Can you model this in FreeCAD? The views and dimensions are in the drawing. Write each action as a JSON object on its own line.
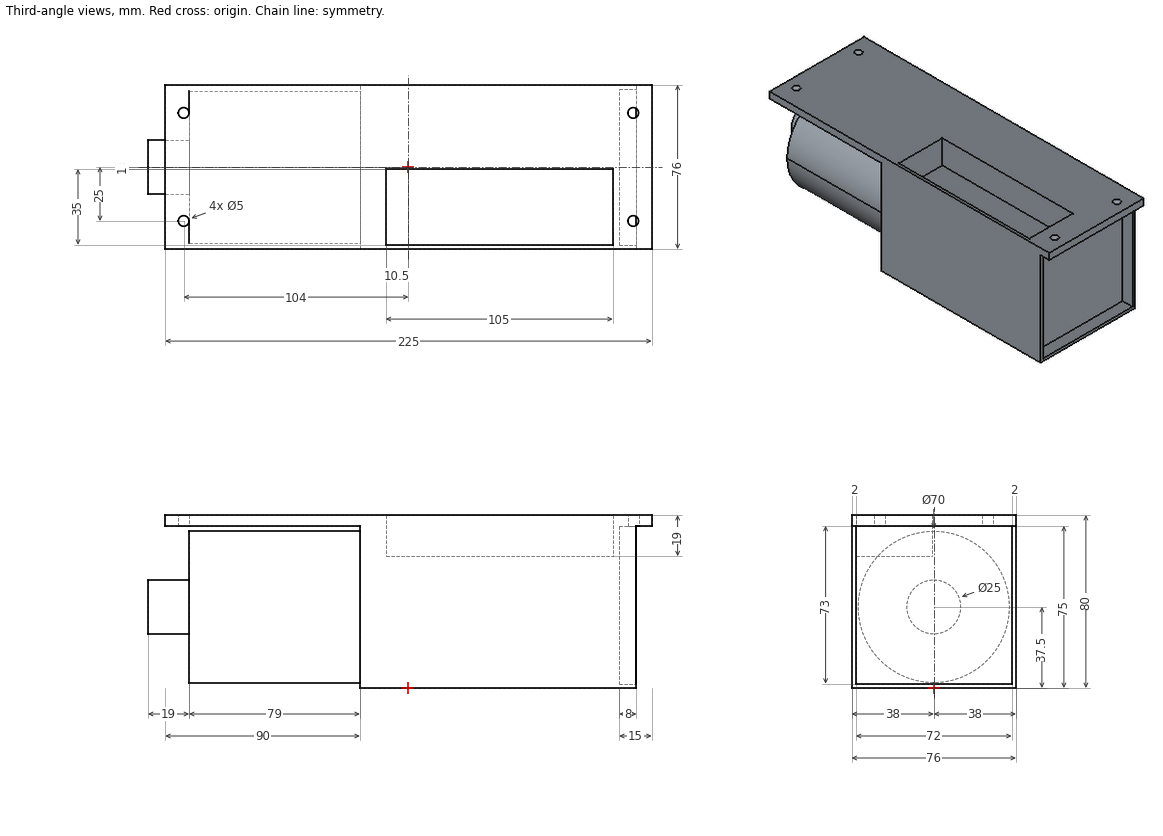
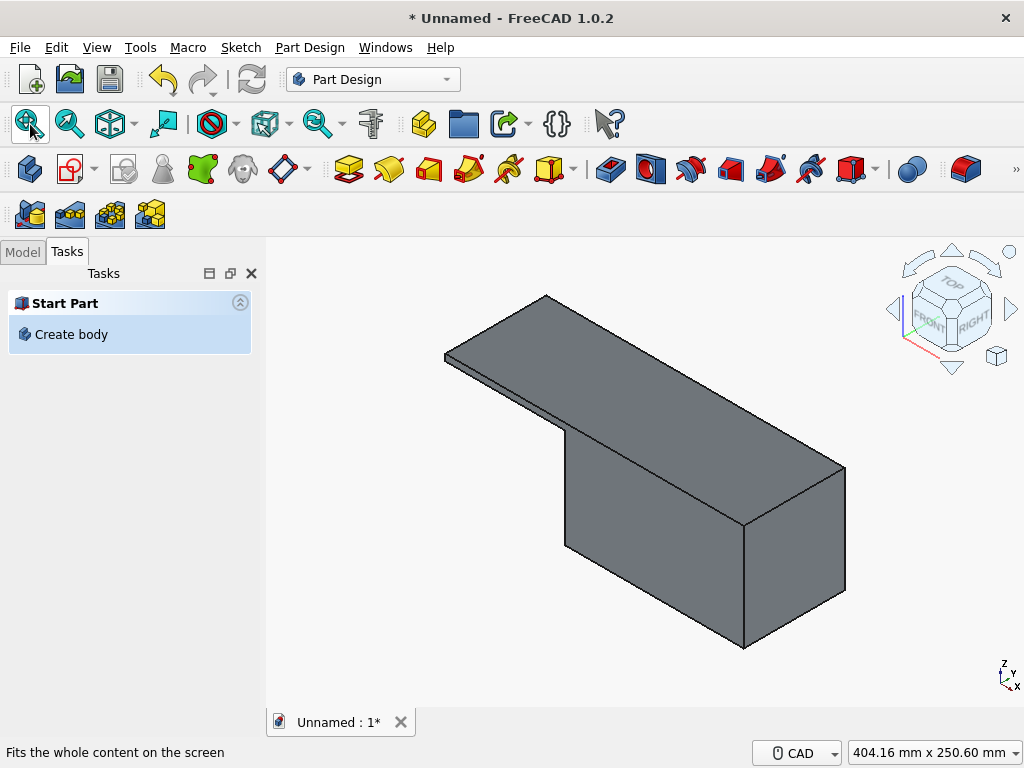
{"action": "left_click", "coordinate": [794, 557]}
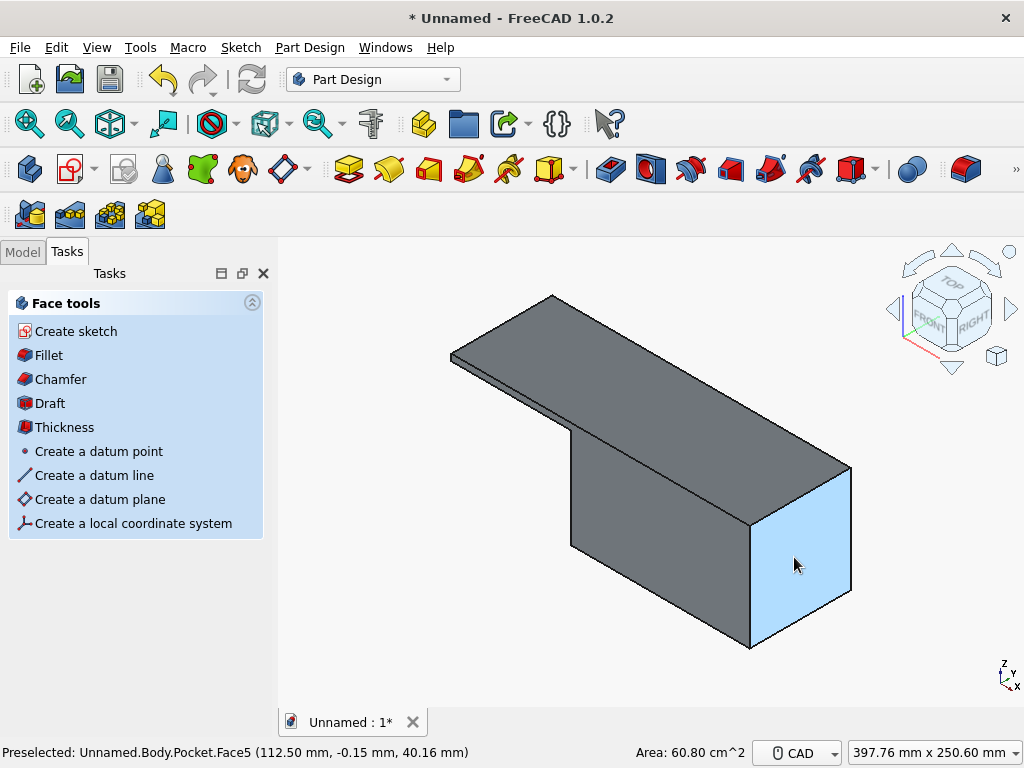
{"action": "left_click", "coordinate": [70, 170]}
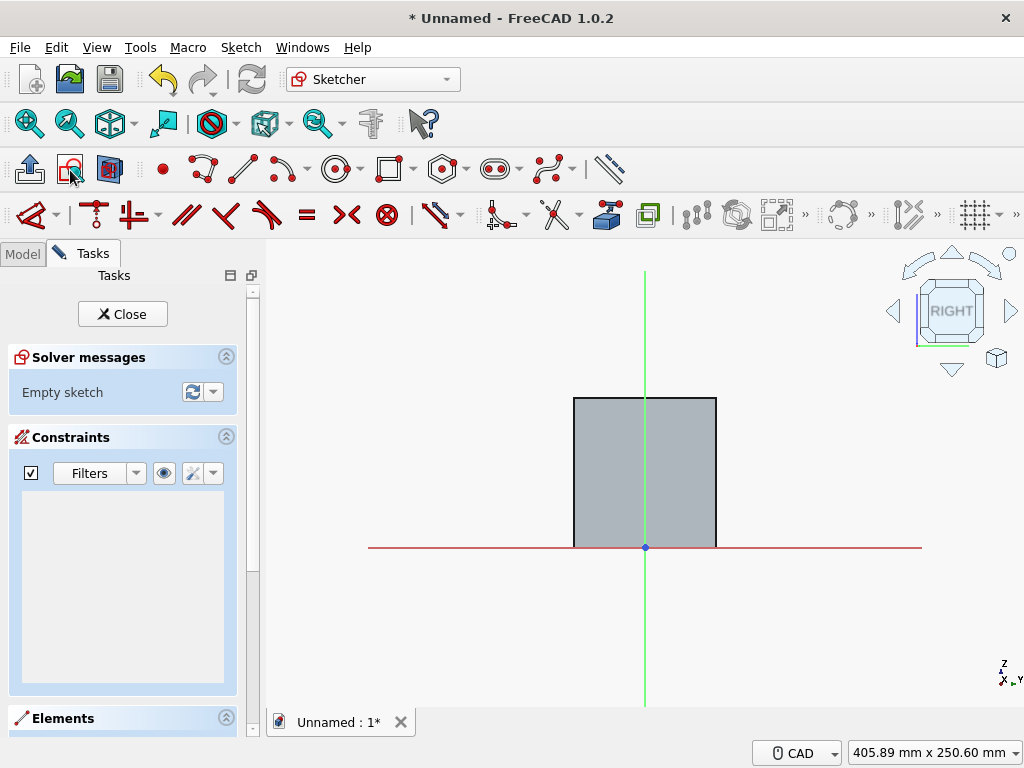
{"action": "scroll", "coordinate": [701, 481], "scroll_direction": "up", "scroll_amount": 4}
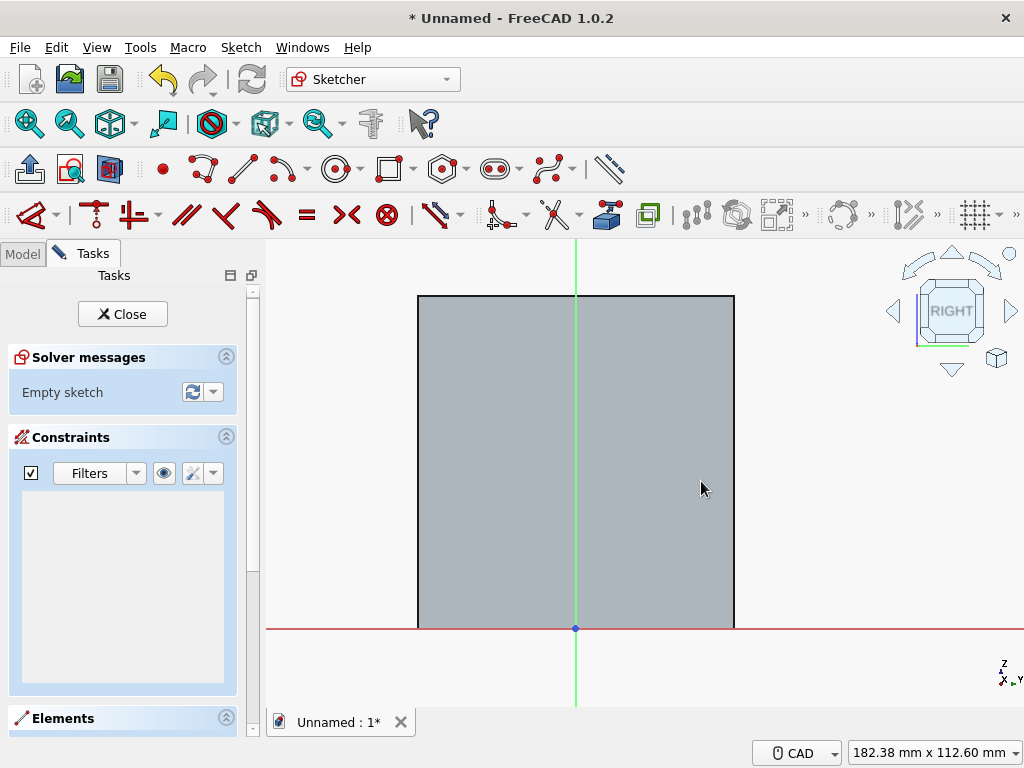
{"action": "key", "text": "g r"}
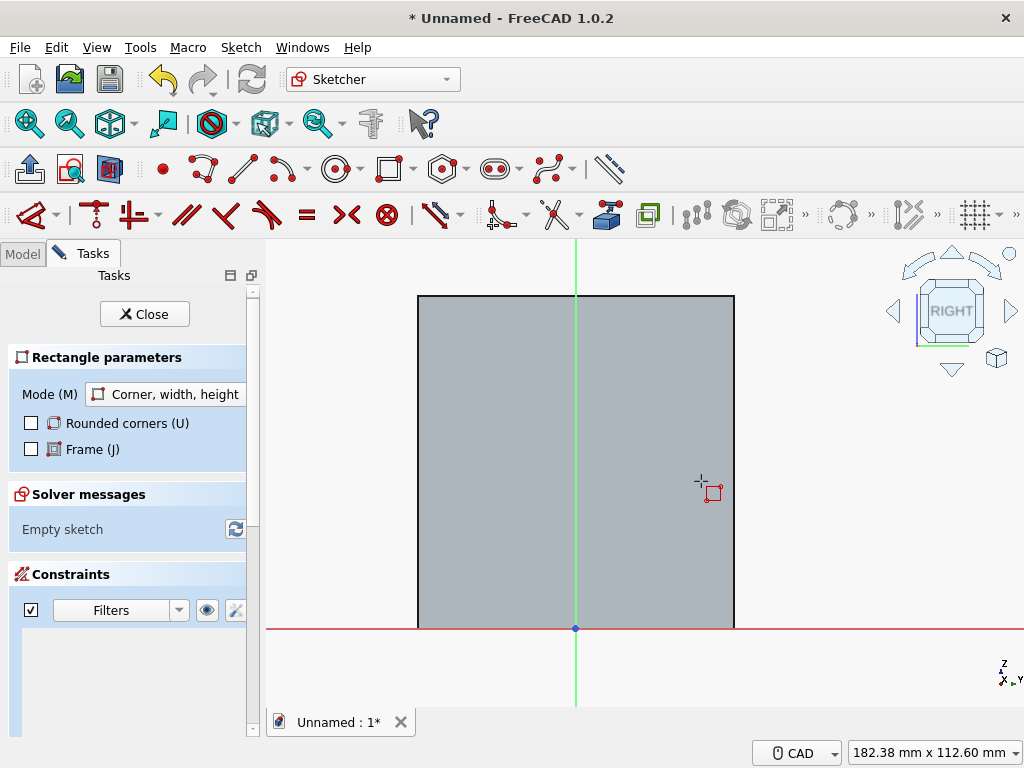
{"action": "left_click", "coordinate": [418, 317]}
{"action": "left_click", "coordinate": [734, 629]}
{"action": "key", "text": "Escape"}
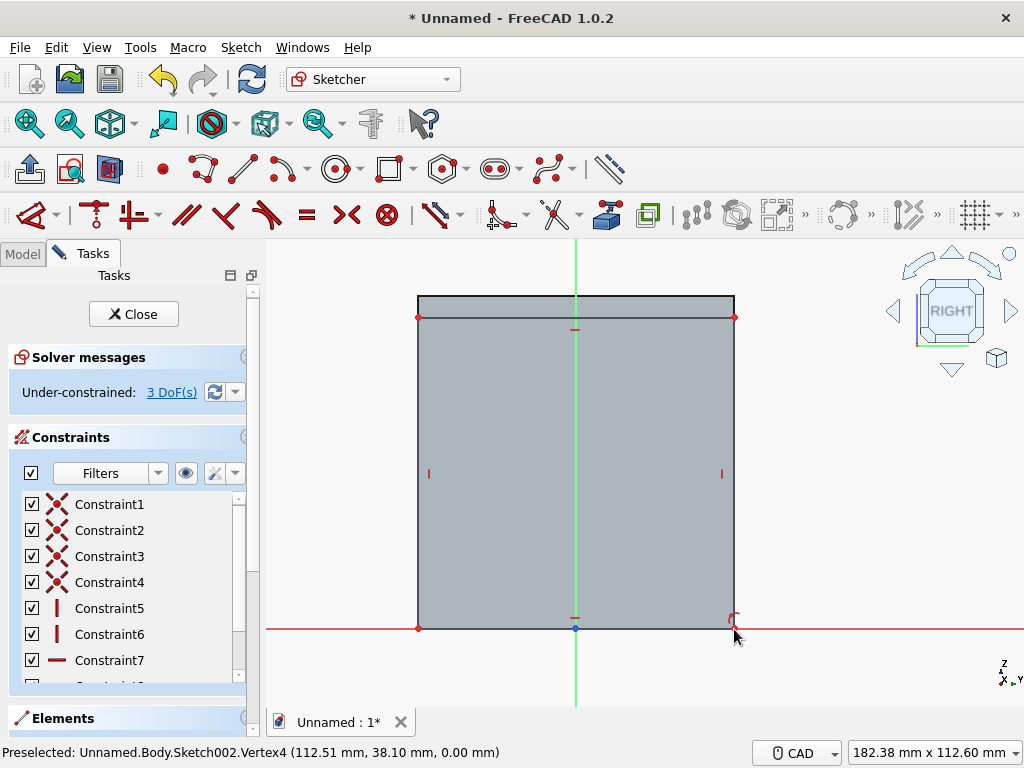
{"action": "key", "text": "d"}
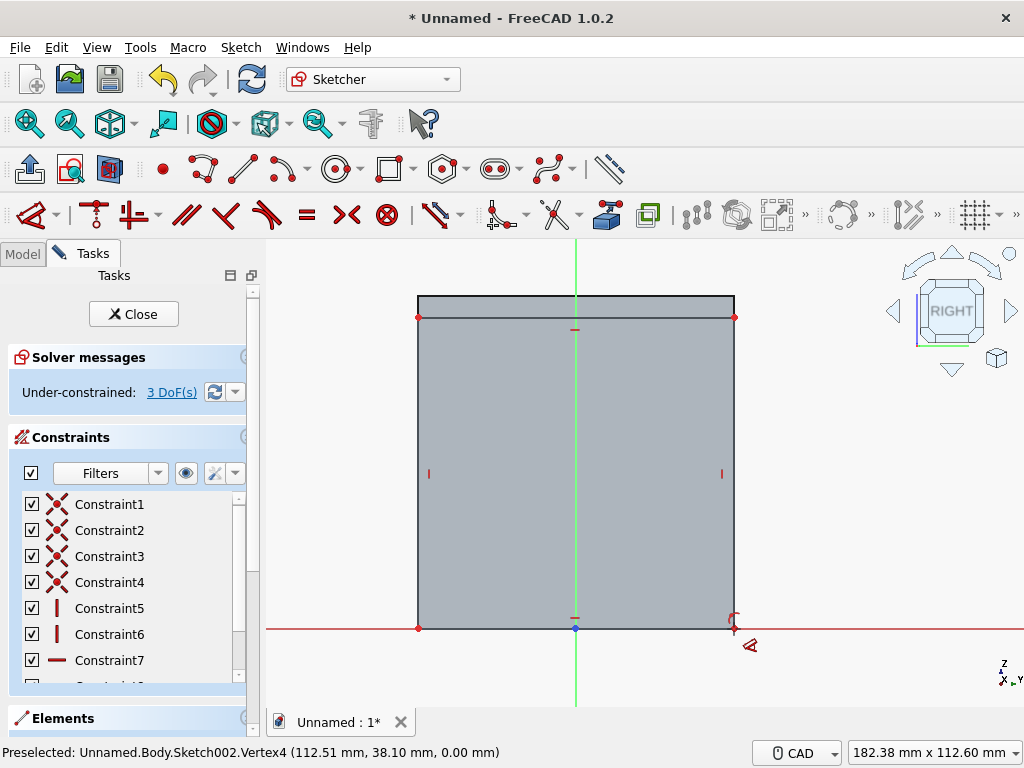
{"action": "left_click", "coordinate": [418, 411]}
{"action": "left_click", "coordinate": [384, 473]}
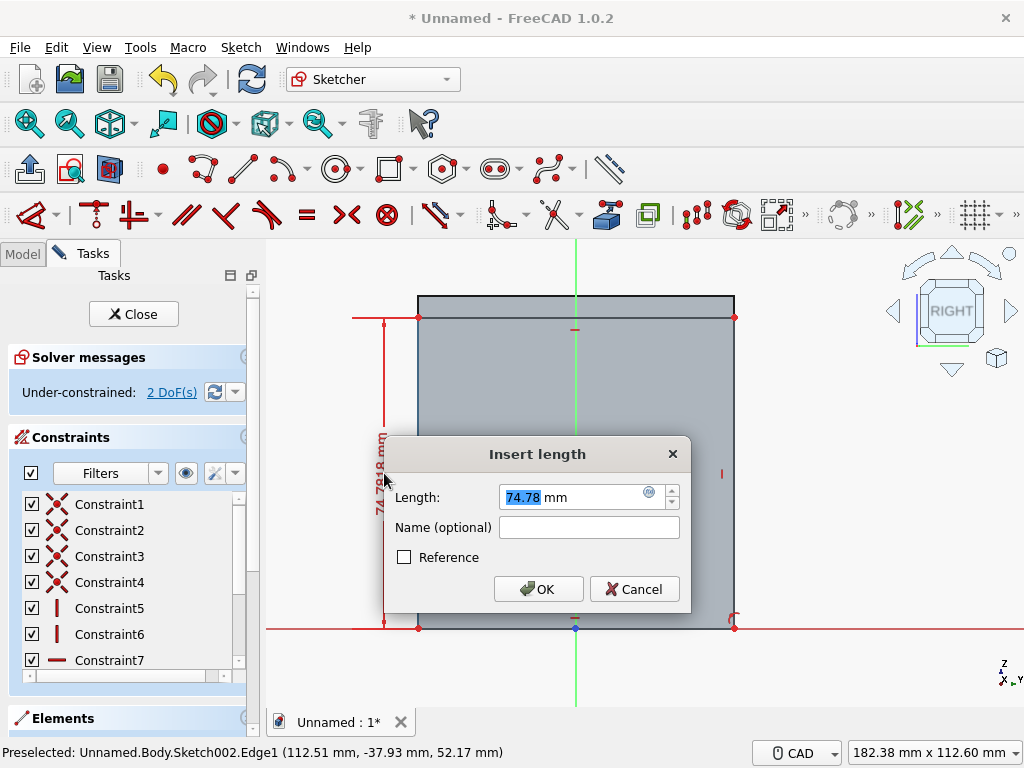
{"action": "type", "text": "75"}
{"action": "key", "text": "Return"}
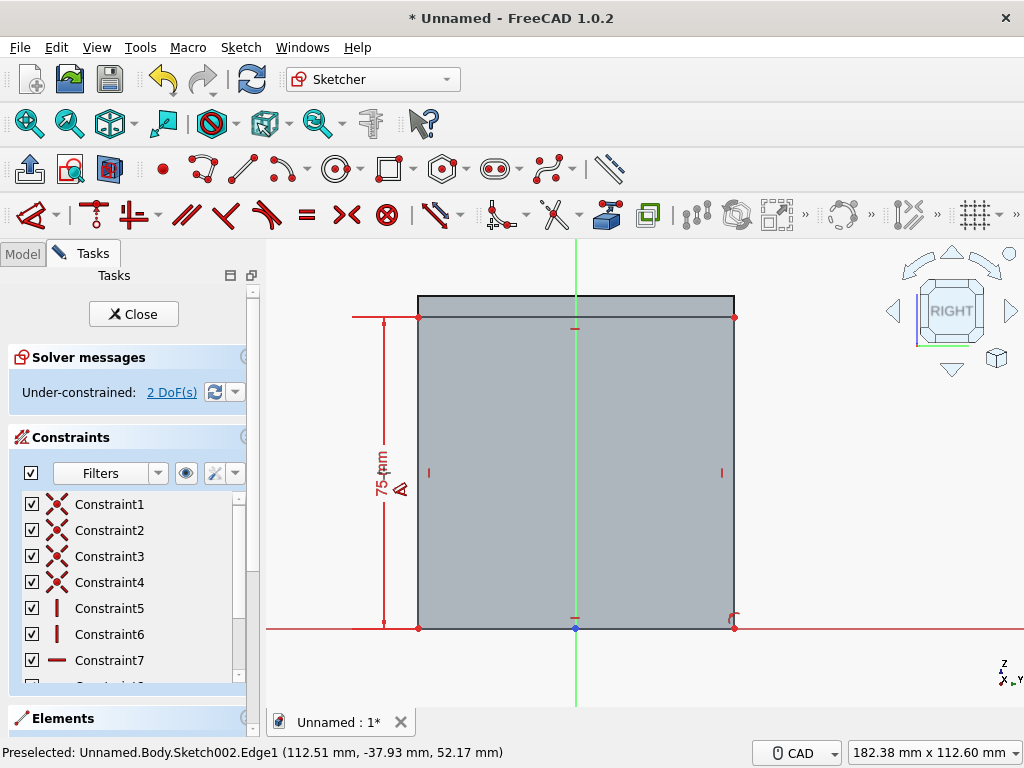
{"action": "left_click", "coordinate": [513, 629]}
{"action": "left_click", "coordinate": [503, 663]}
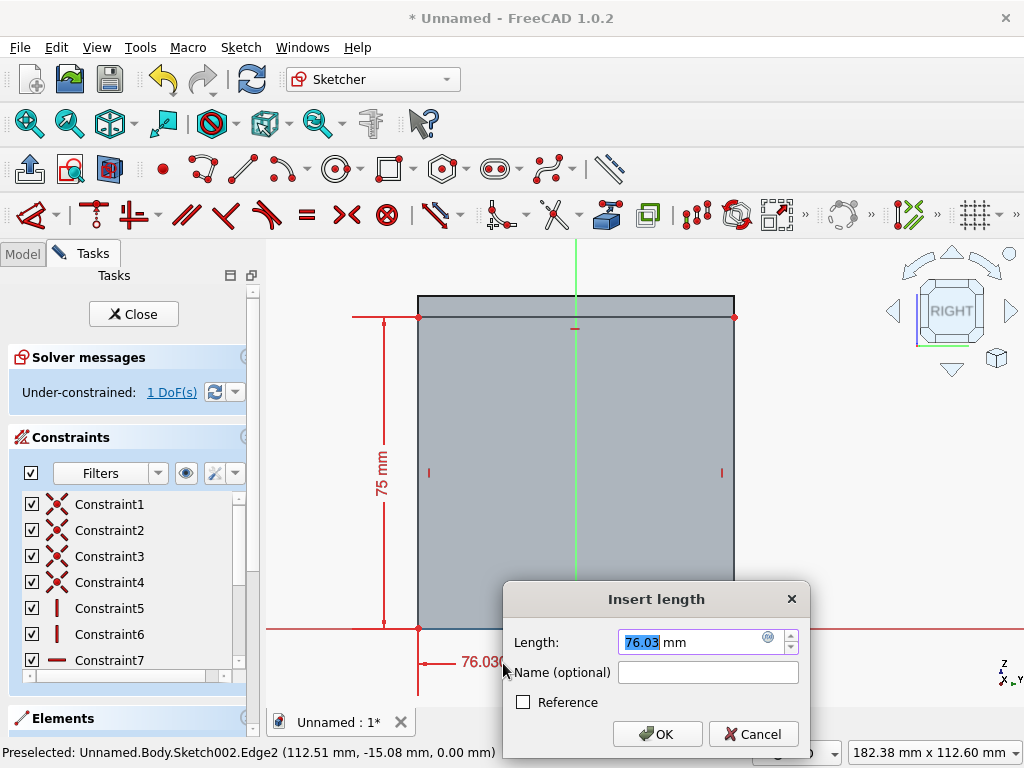
{"action": "type", "text": "76"}
{"action": "key", "text": "Return"}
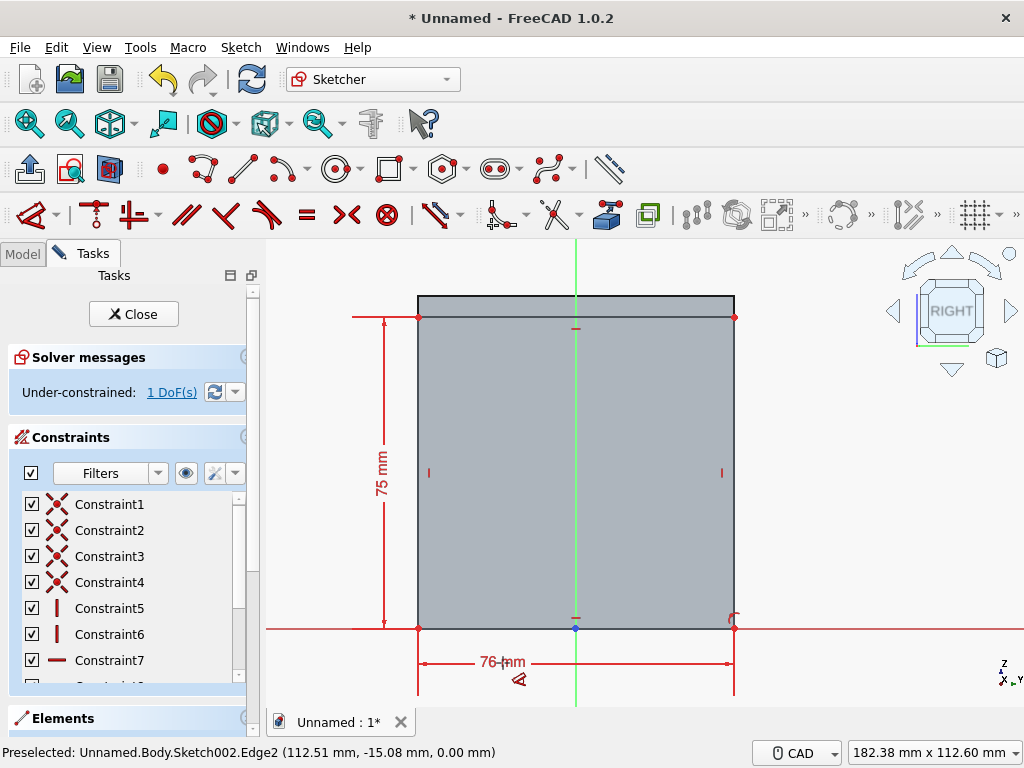
{"action": "left_click", "coordinate": [418, 317]}
{"action": "left_click", "coordinate": [497, 283]}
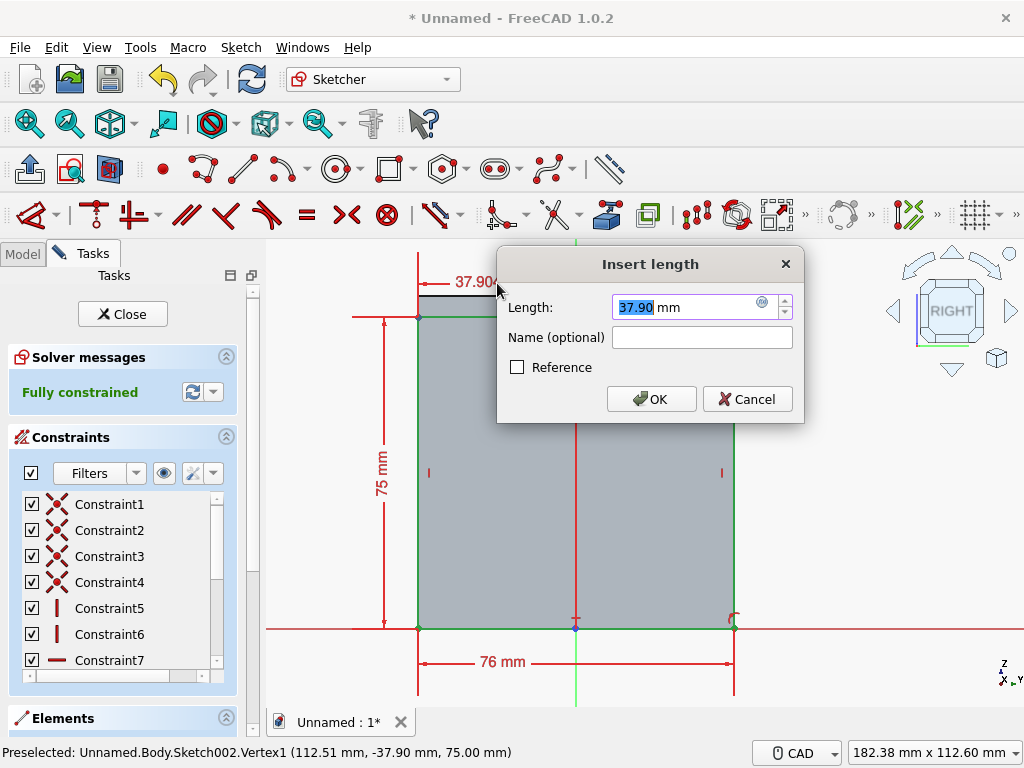
{"action": "type", "text": "38"}
{"action": "key", "text": "Return"}
{"action": "key", "text": "Escape"}